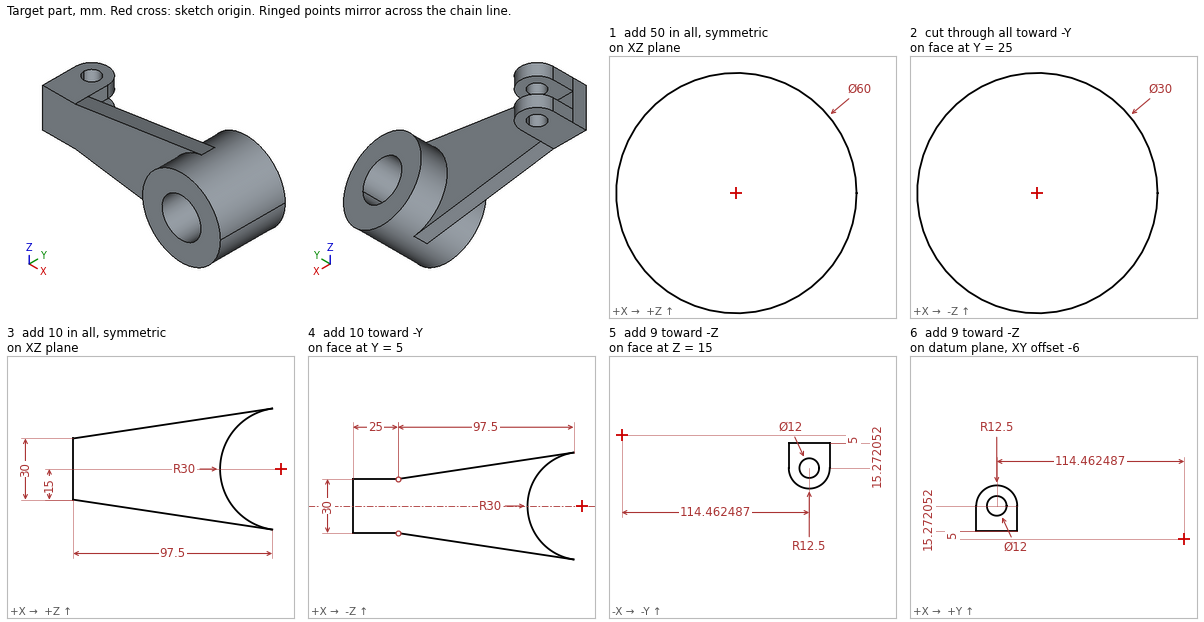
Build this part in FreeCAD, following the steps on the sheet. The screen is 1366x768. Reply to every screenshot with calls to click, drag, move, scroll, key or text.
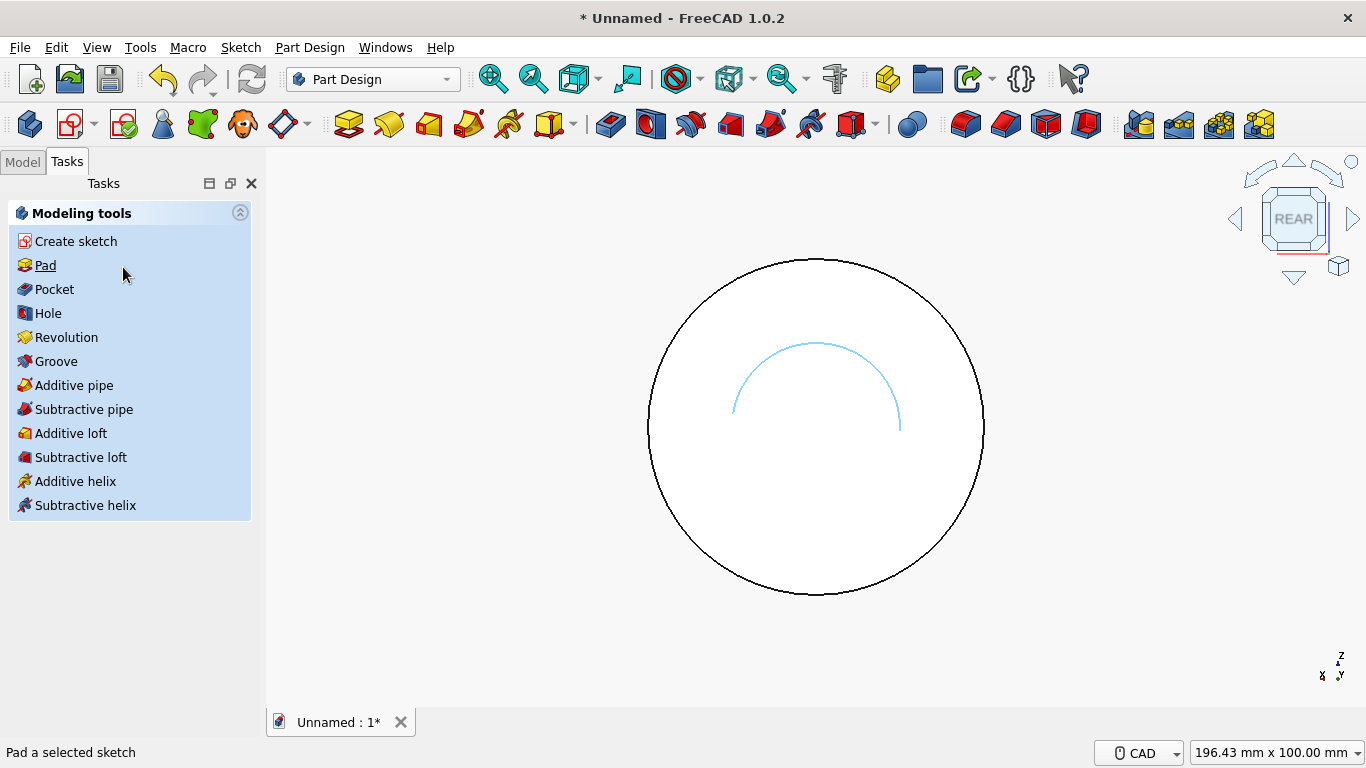
click(612, 124)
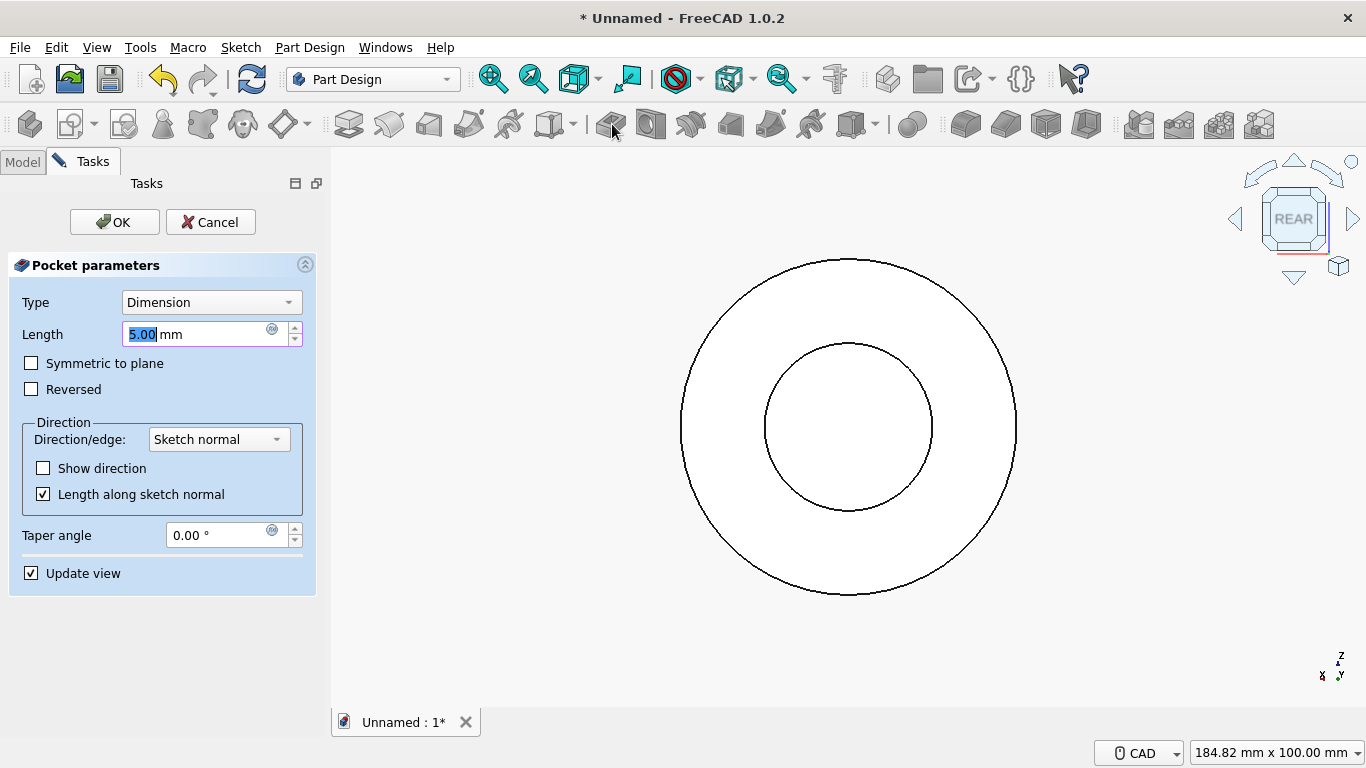
click(212, 302)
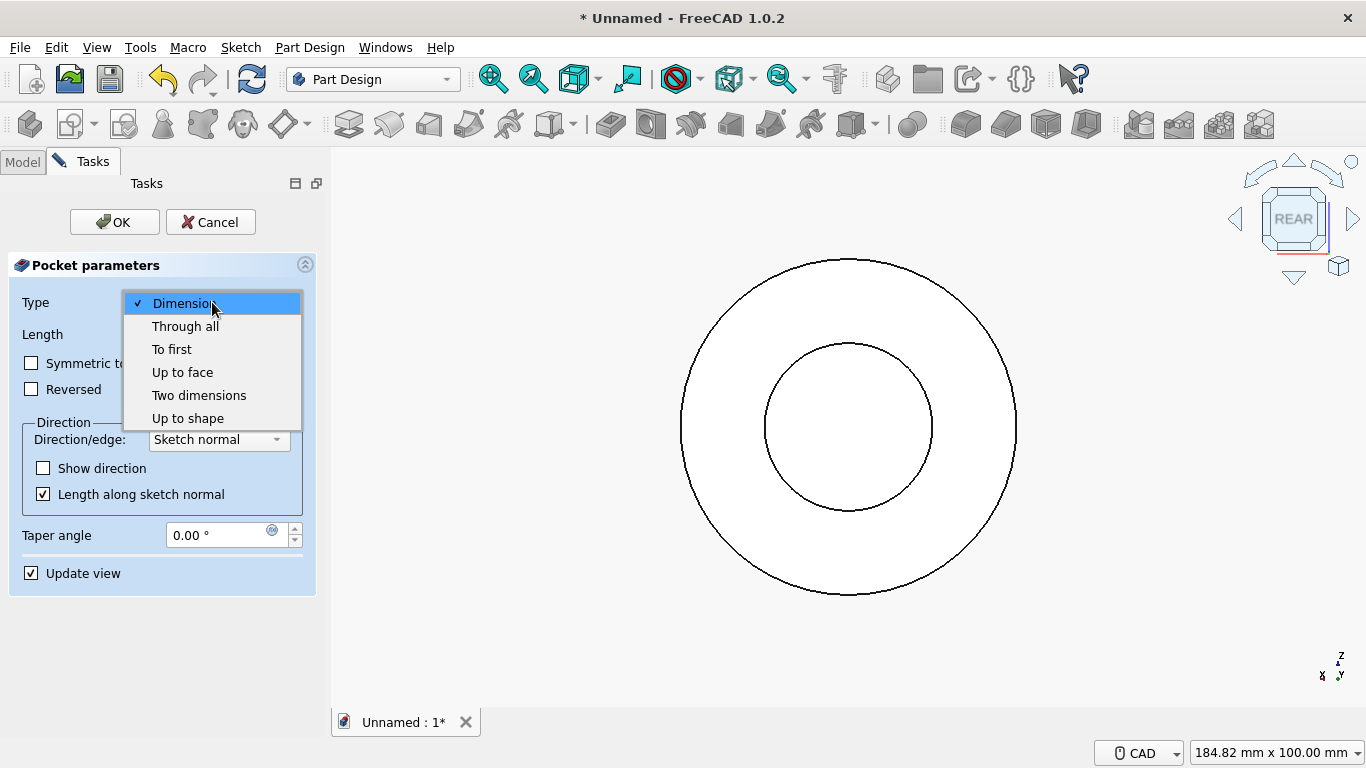
click(212, 326)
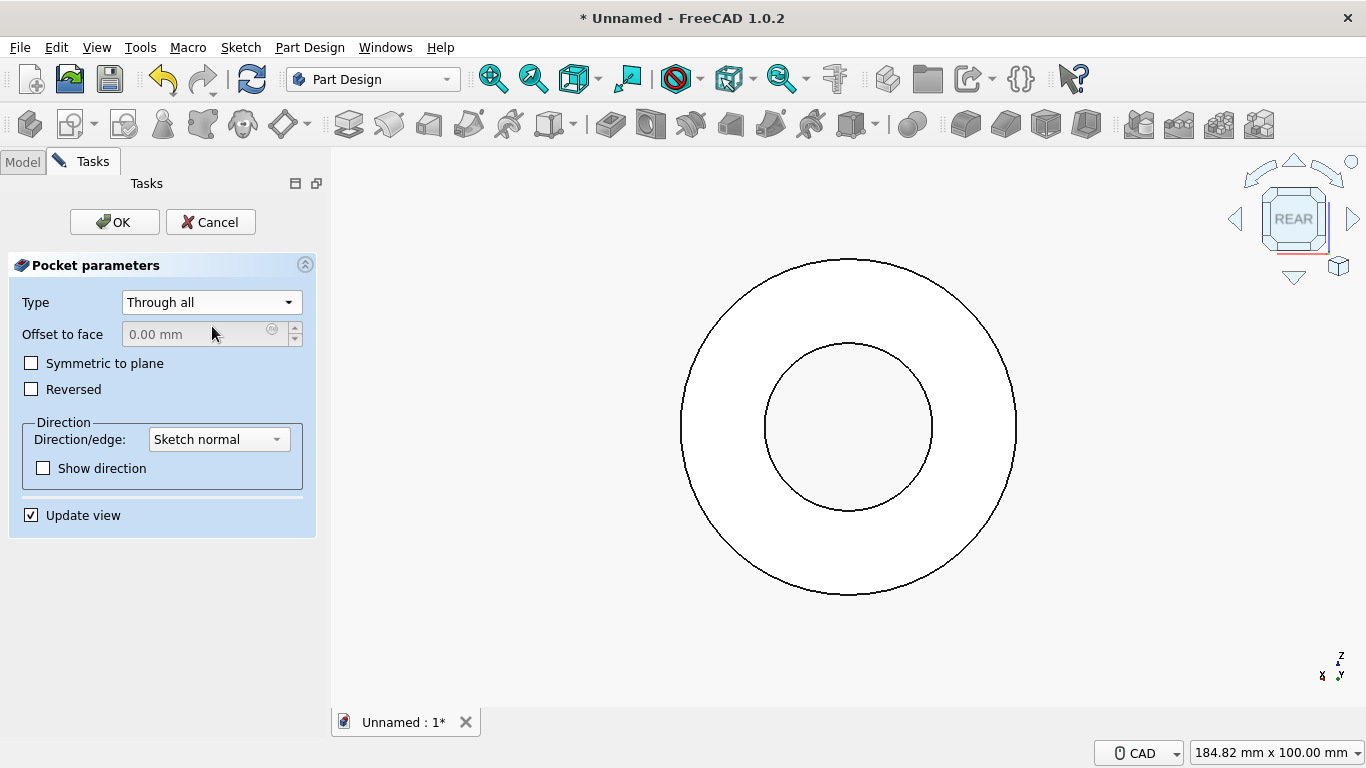
click(115, 222)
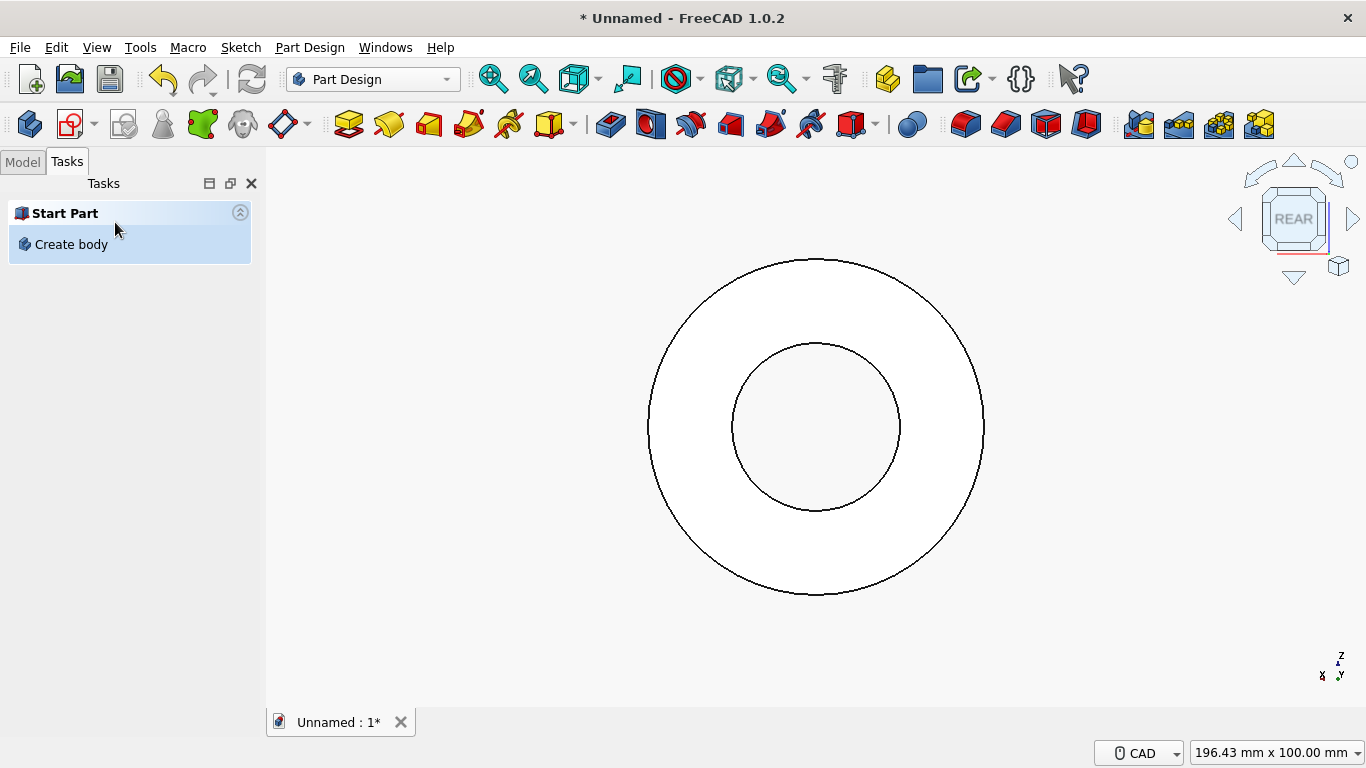
click(70, 124)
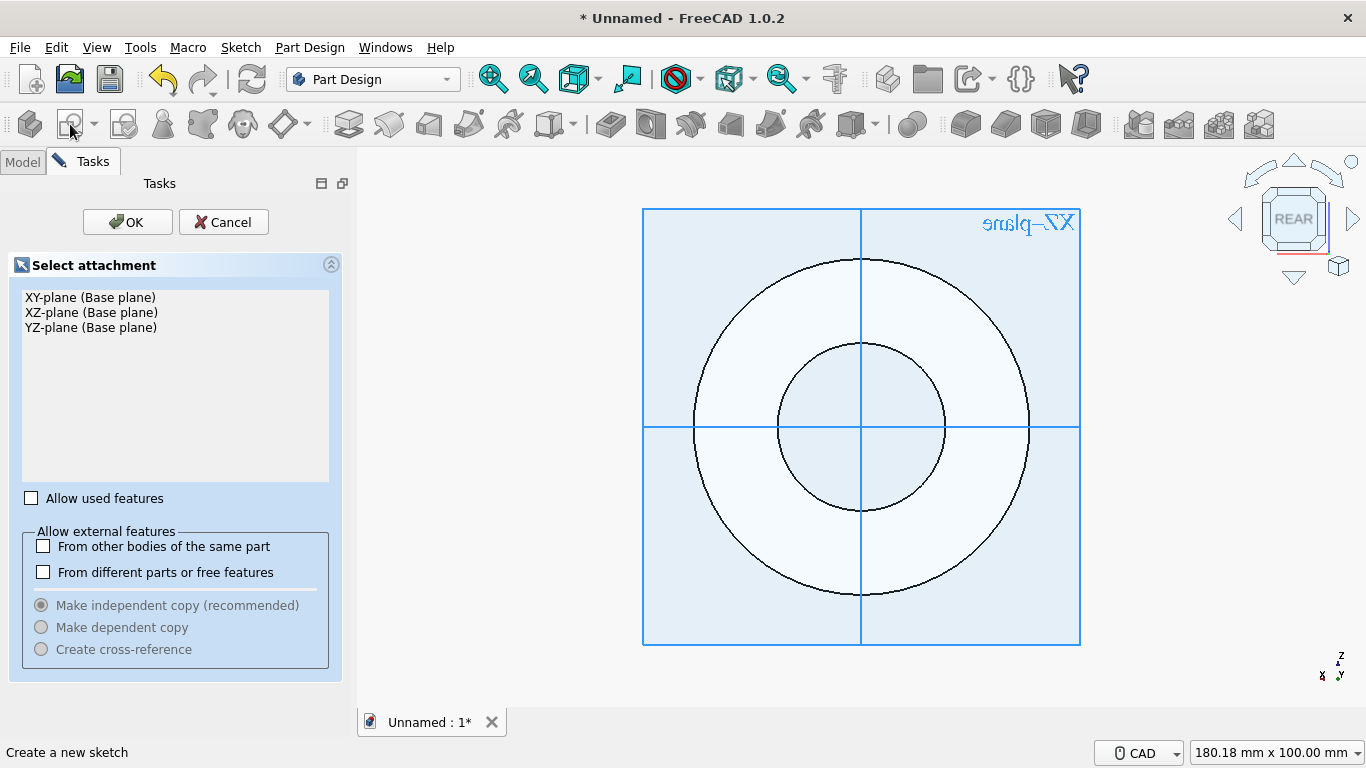
click(82, 312)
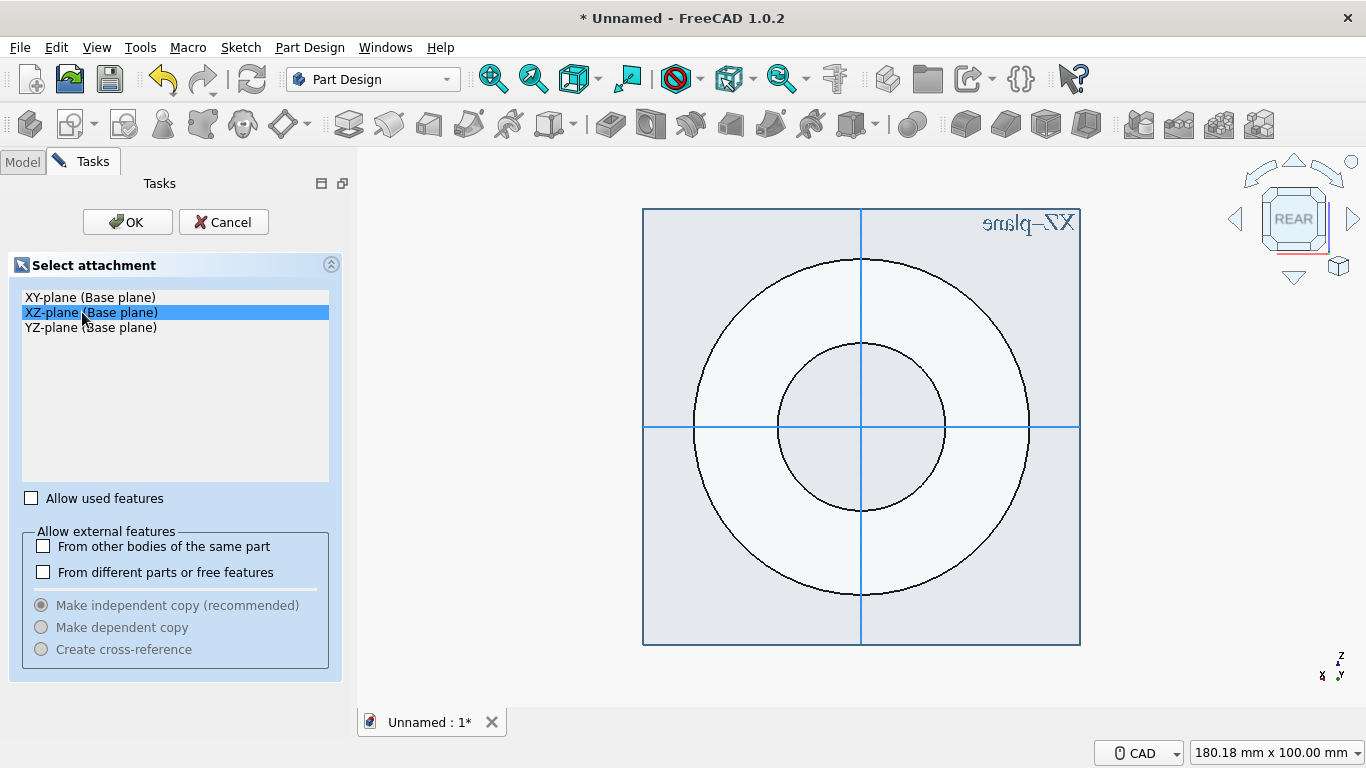
click(128, 222)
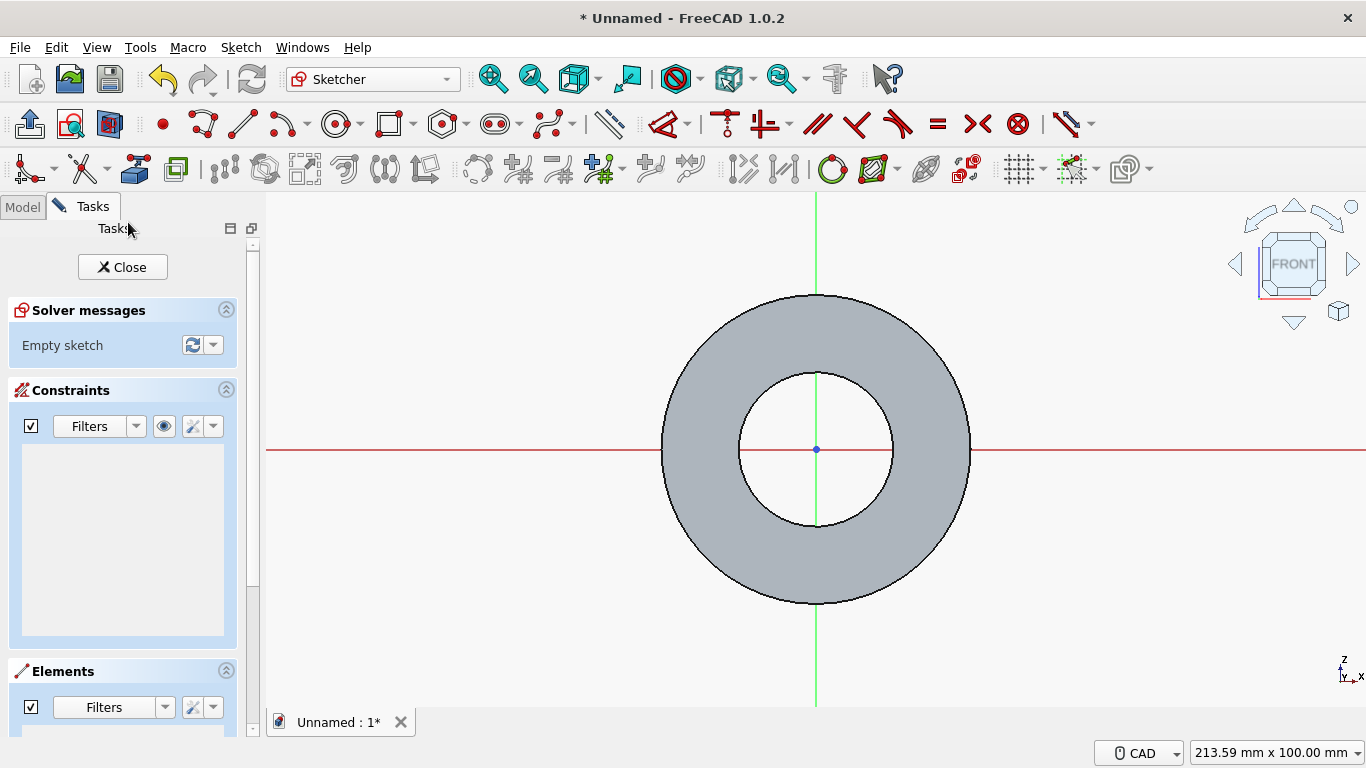
key(q)
key(s)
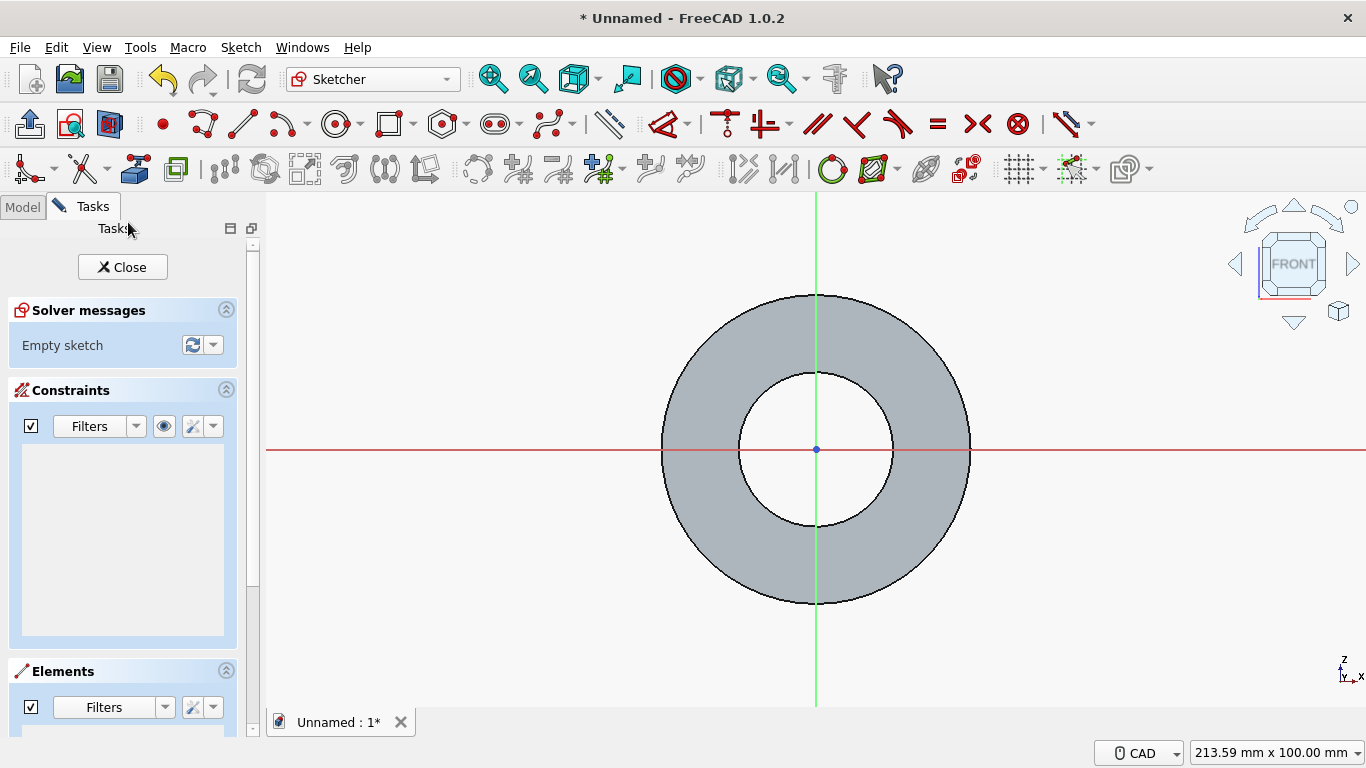
scroll(1201, 449, down, 1)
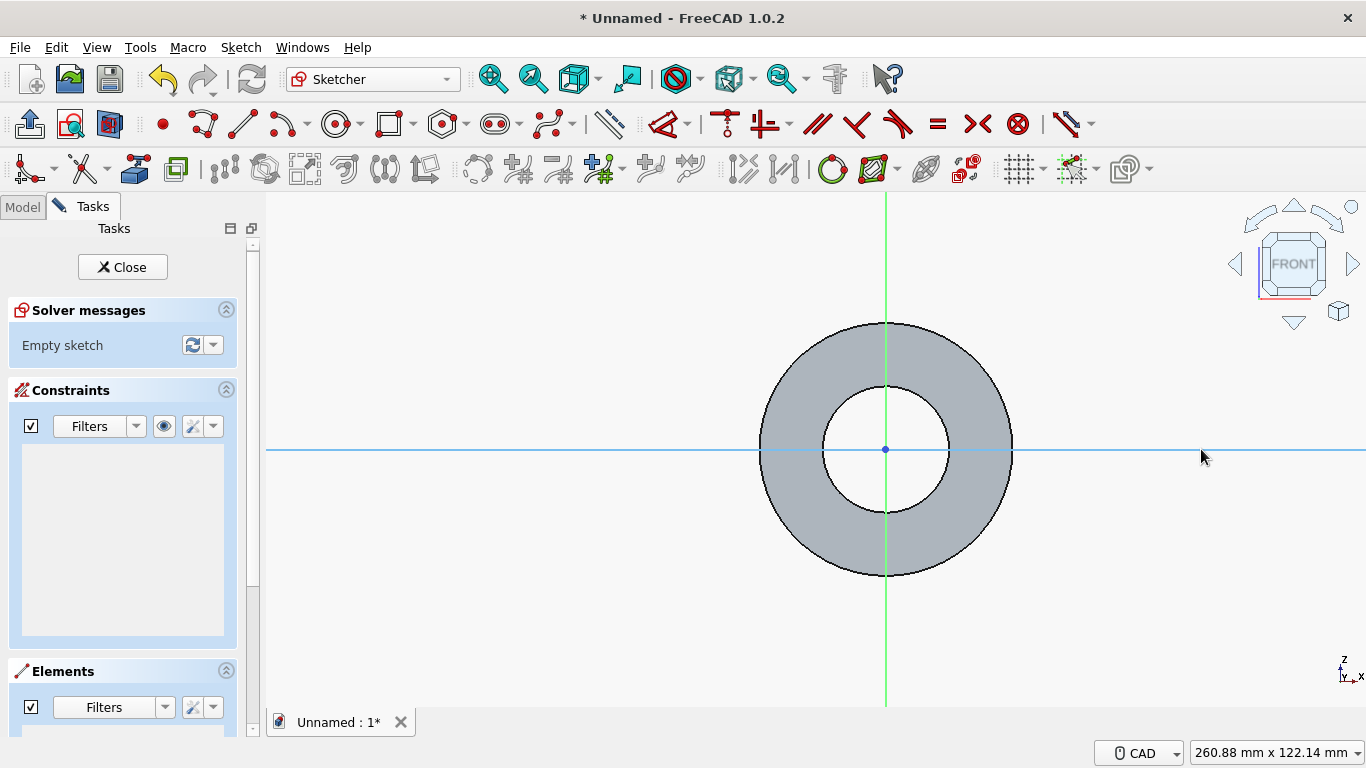
click(204, 124)